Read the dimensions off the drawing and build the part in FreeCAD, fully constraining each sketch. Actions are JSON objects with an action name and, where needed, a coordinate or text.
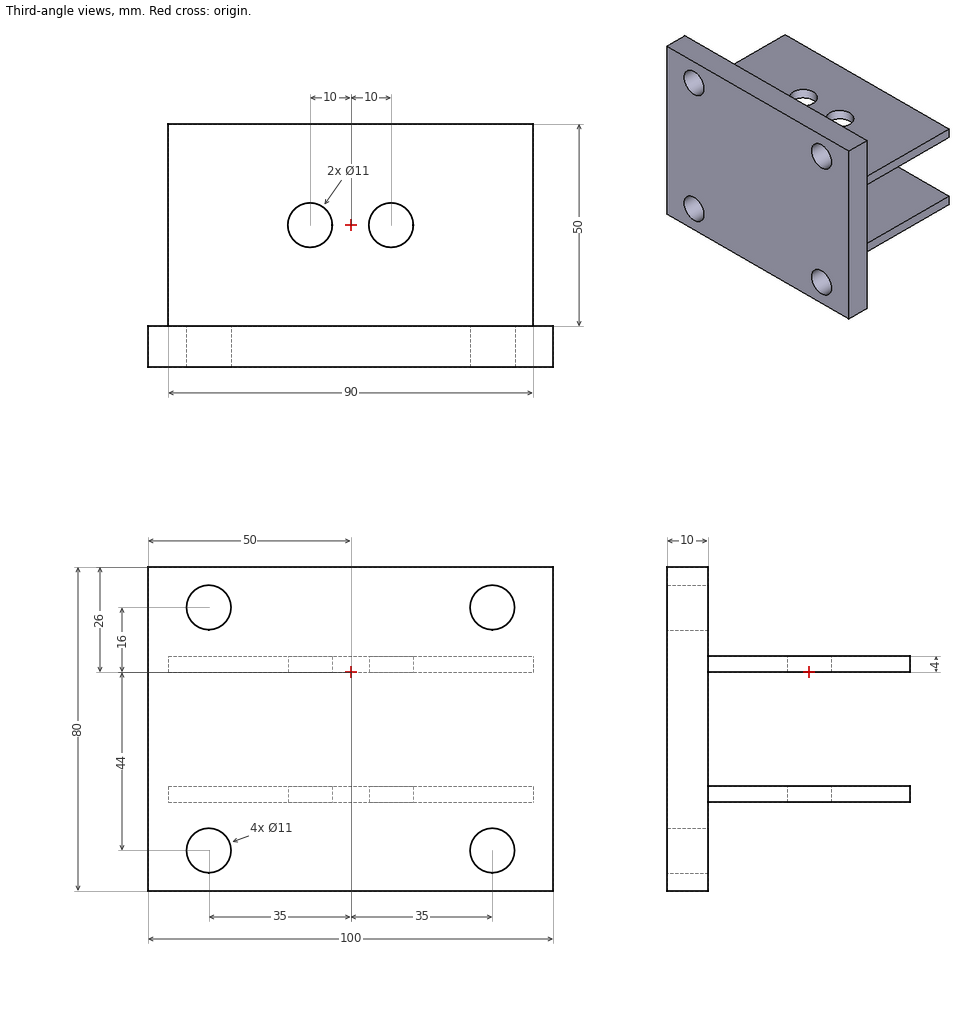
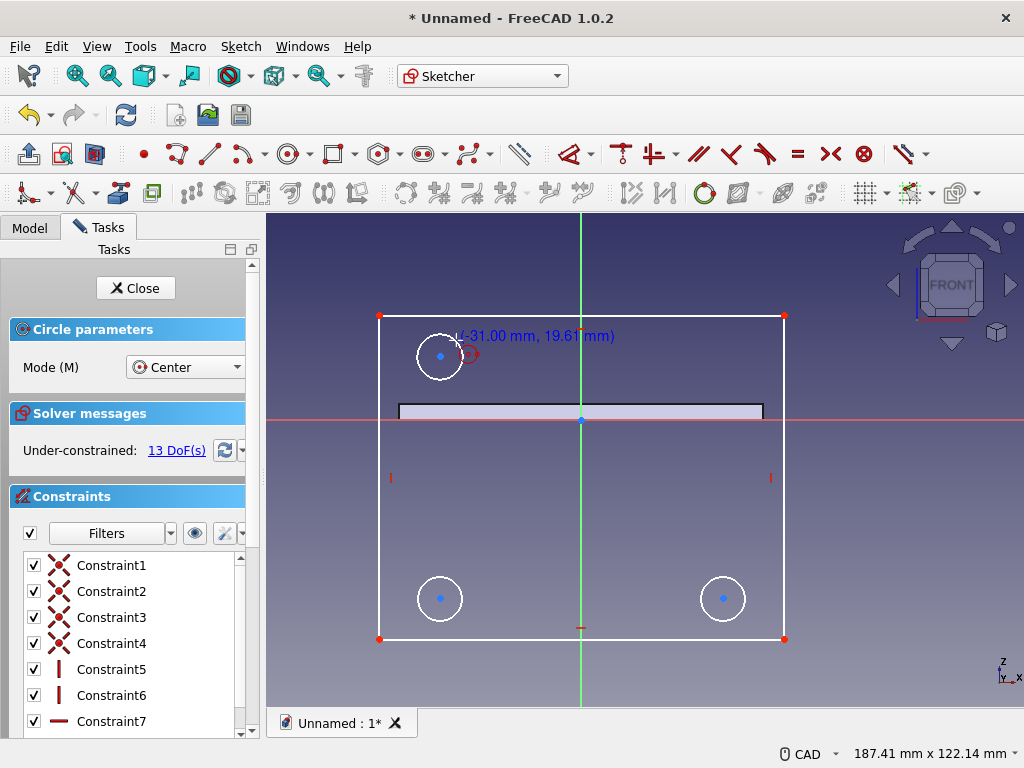
{"action": "left_click", "coordinate": [723, 356]}
{"action": "left_click", "coordinate": [739, 340]}
{"action": "key", "text": "Escape"}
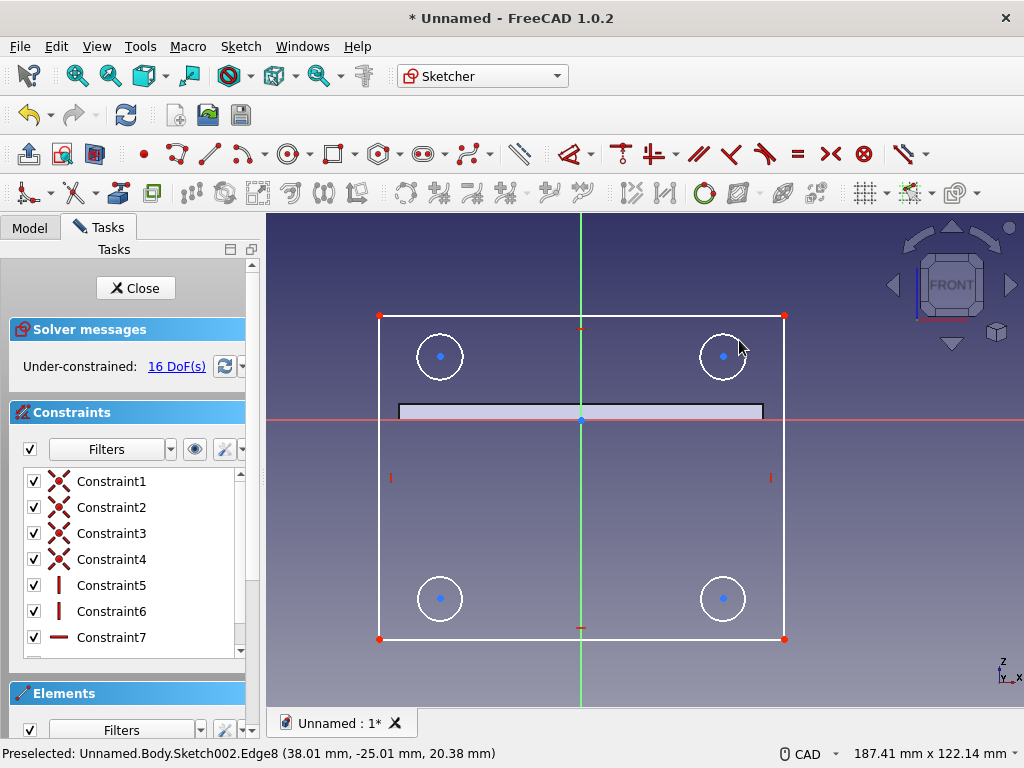
{"action": "left_click", "coordinate": [455, 583]}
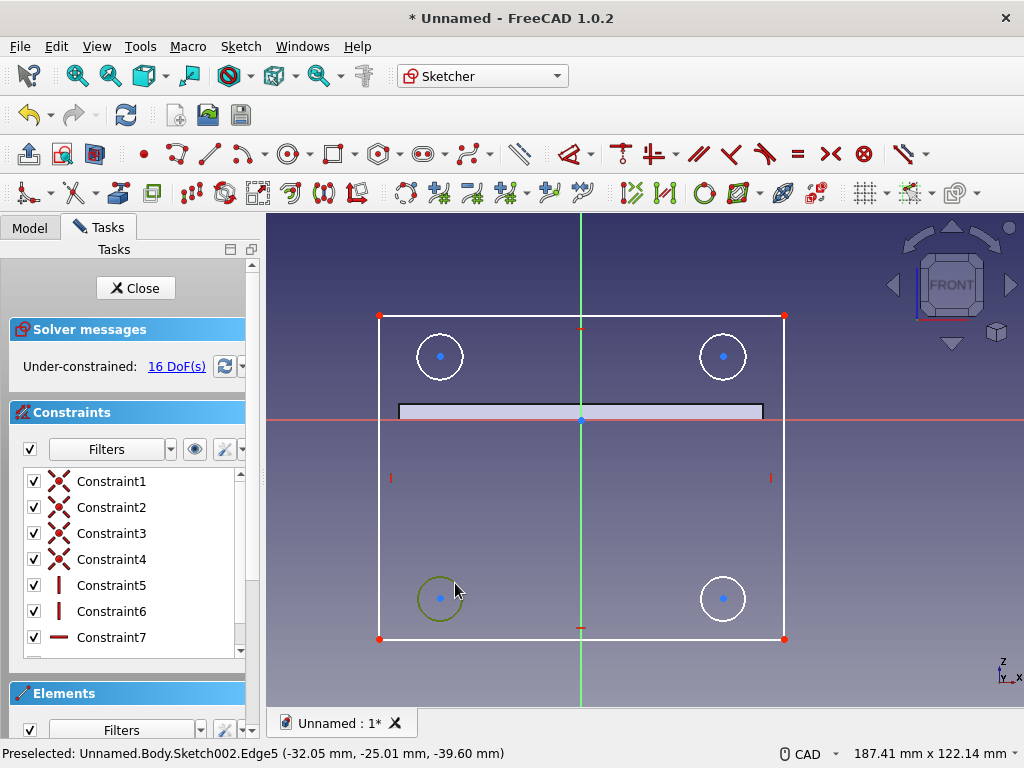
{"action": "left_click", "coordinate": [738, 583]}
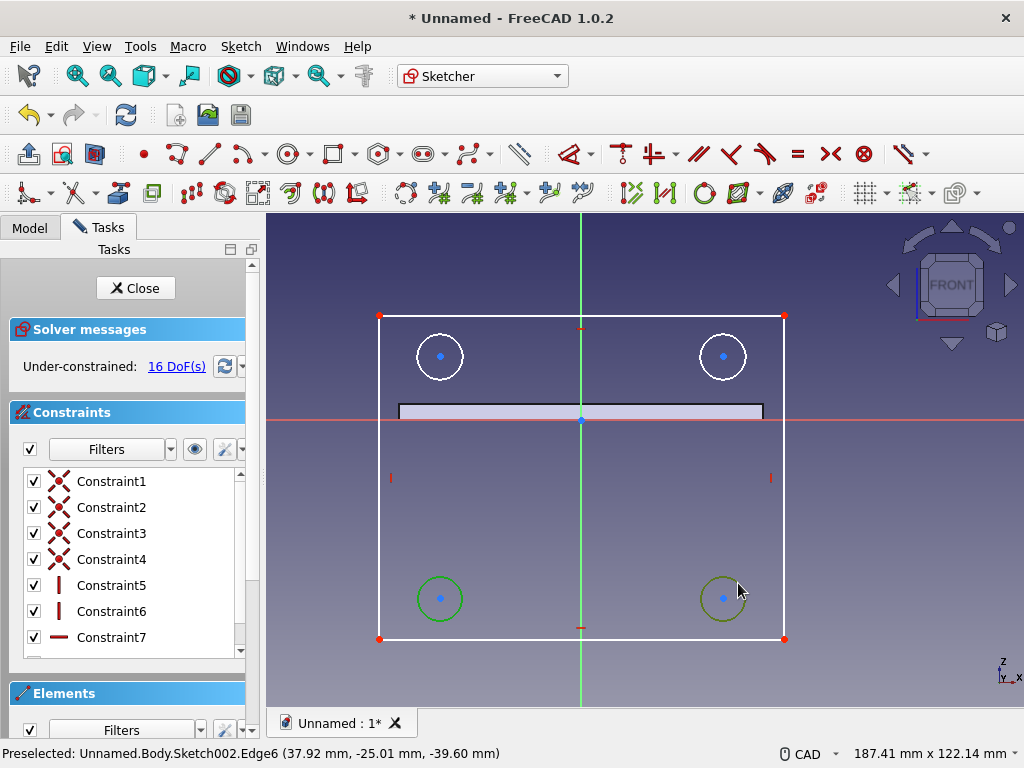
{"action": "left_click", "coordinate": [456, 341]}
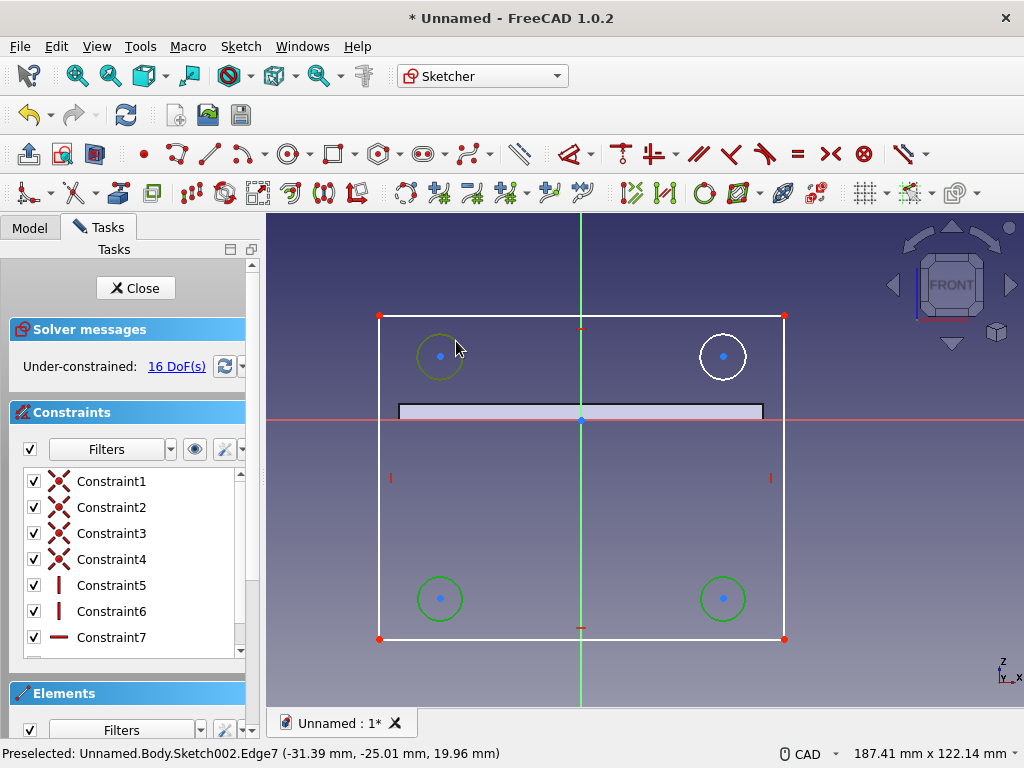
{"action": "left_click", "coordinate": [739, 341]}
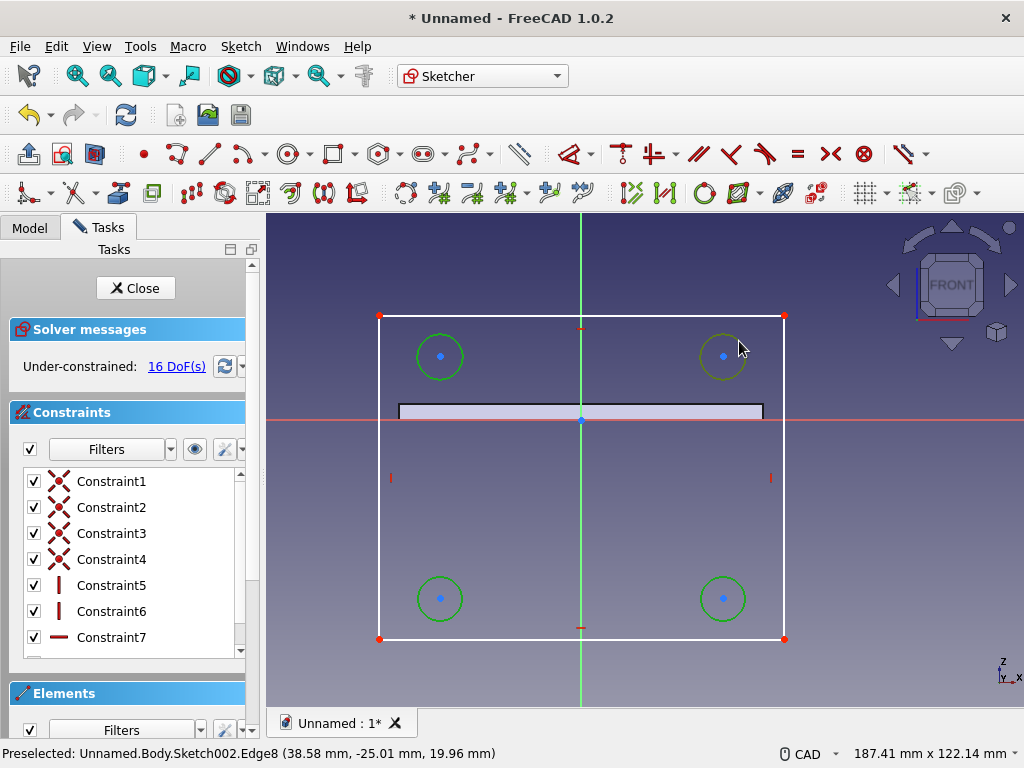
{"action": "key", "text": "e"}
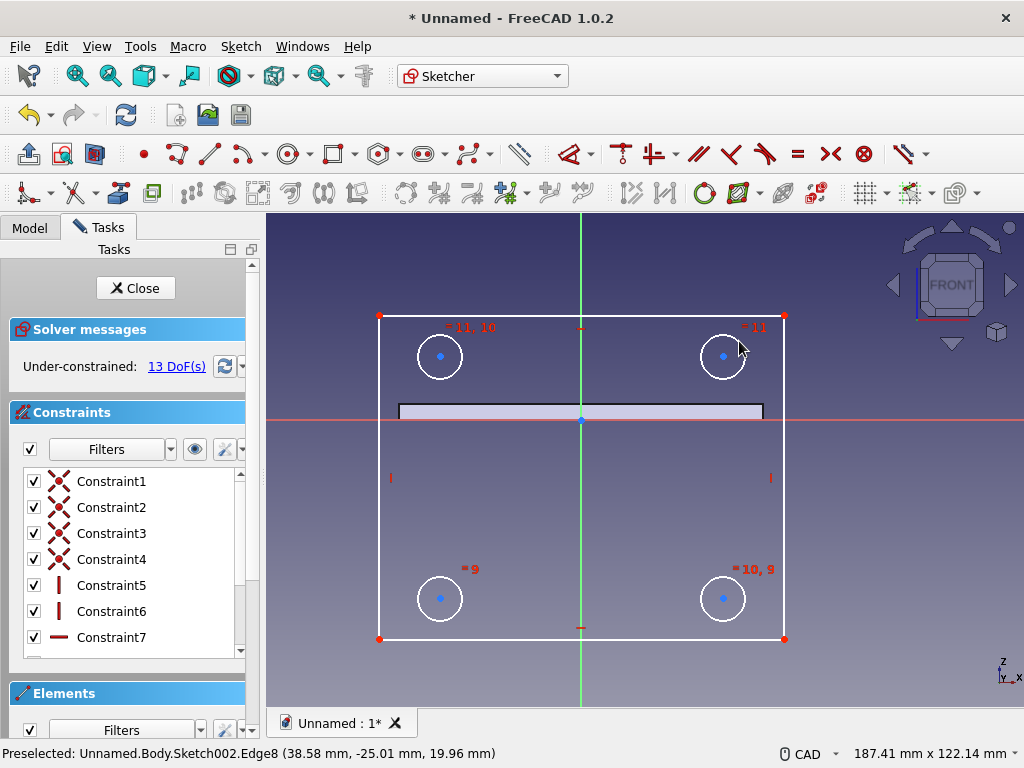
{"action": "left_click", "coordinate": [440, 599]}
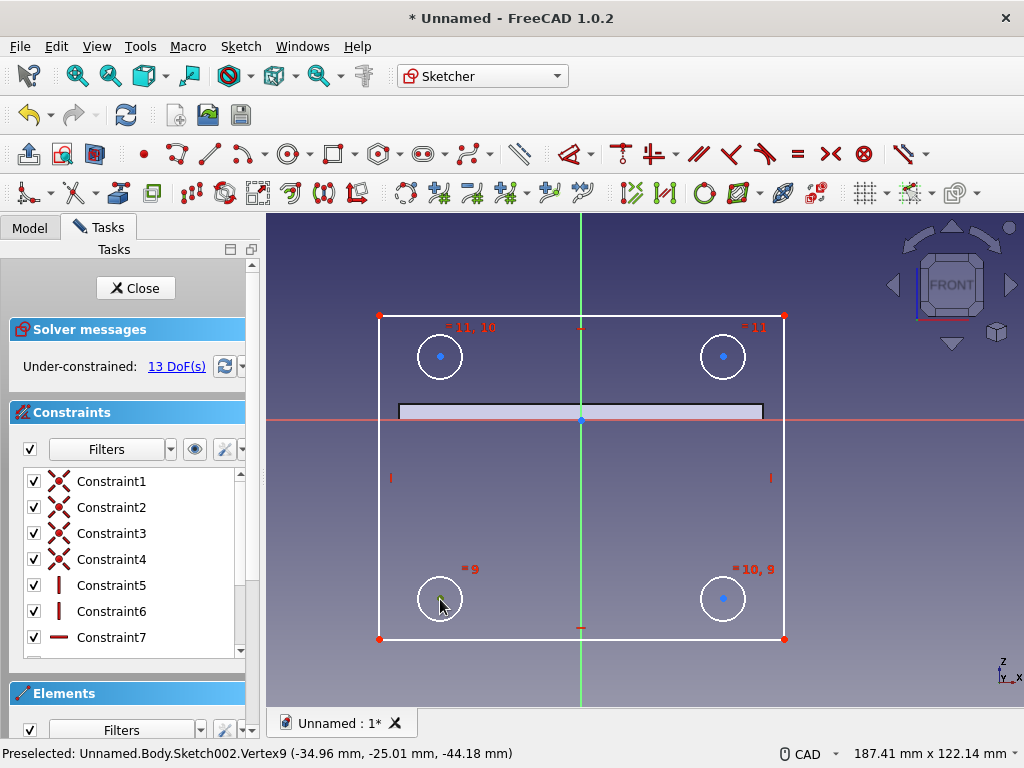
{"action": "left_click", "coordinate": [723, 599]}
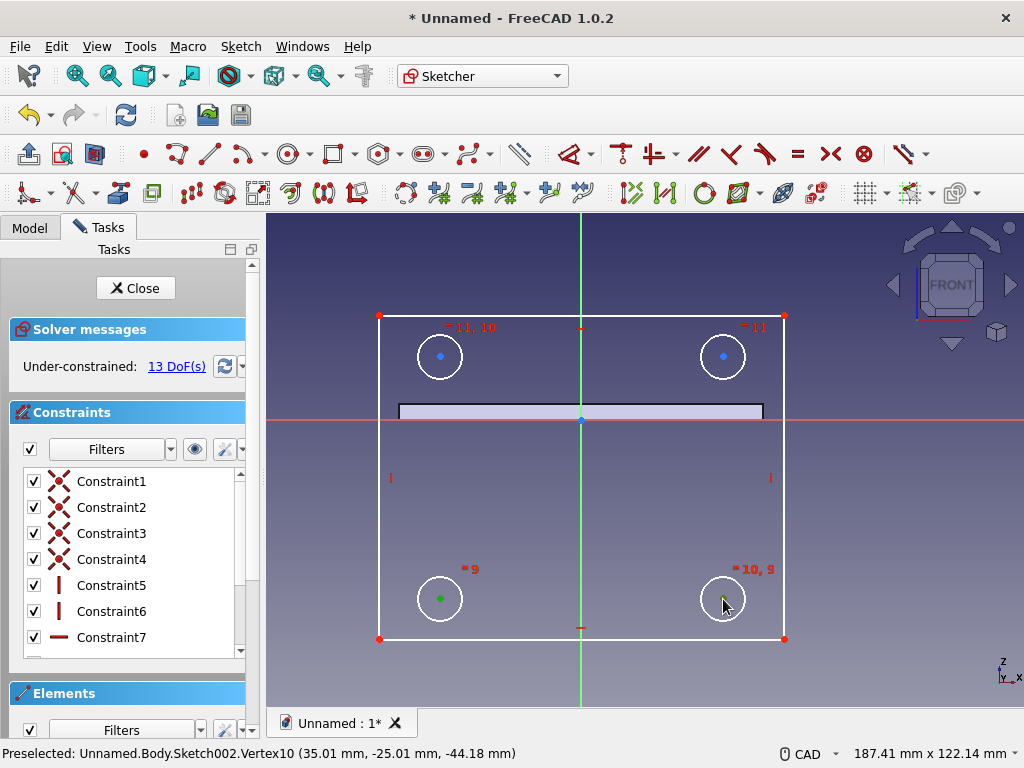
{"action": "key", "text": "h"}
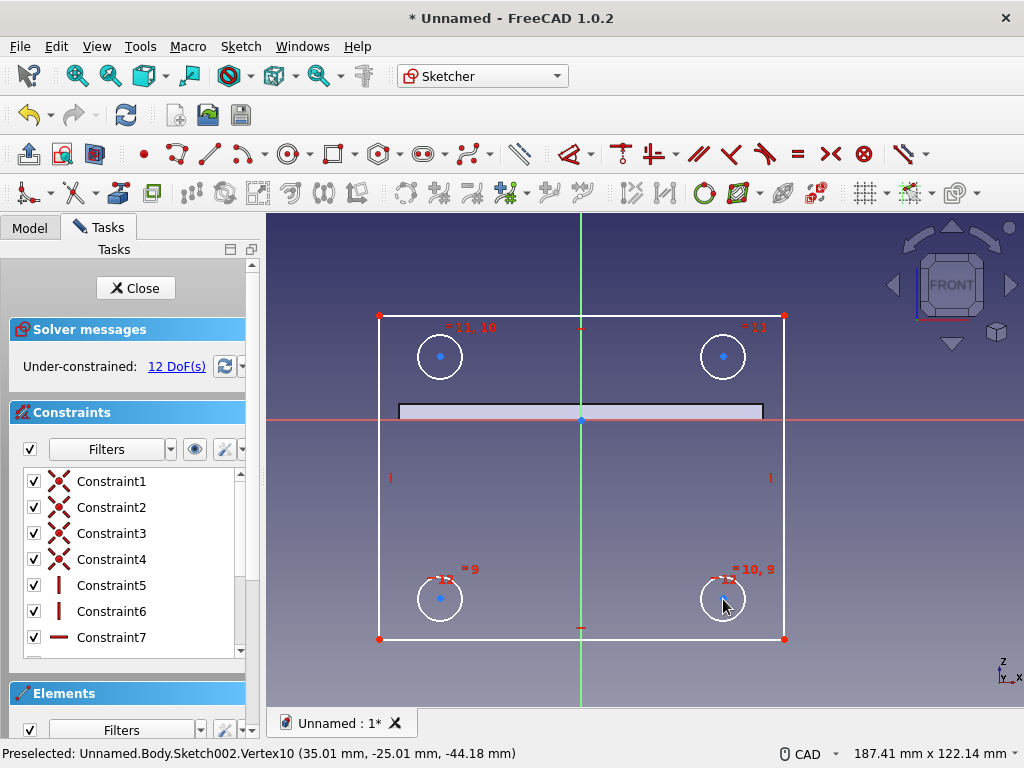
{"action": "left_click", "coordinate": [440, 599]}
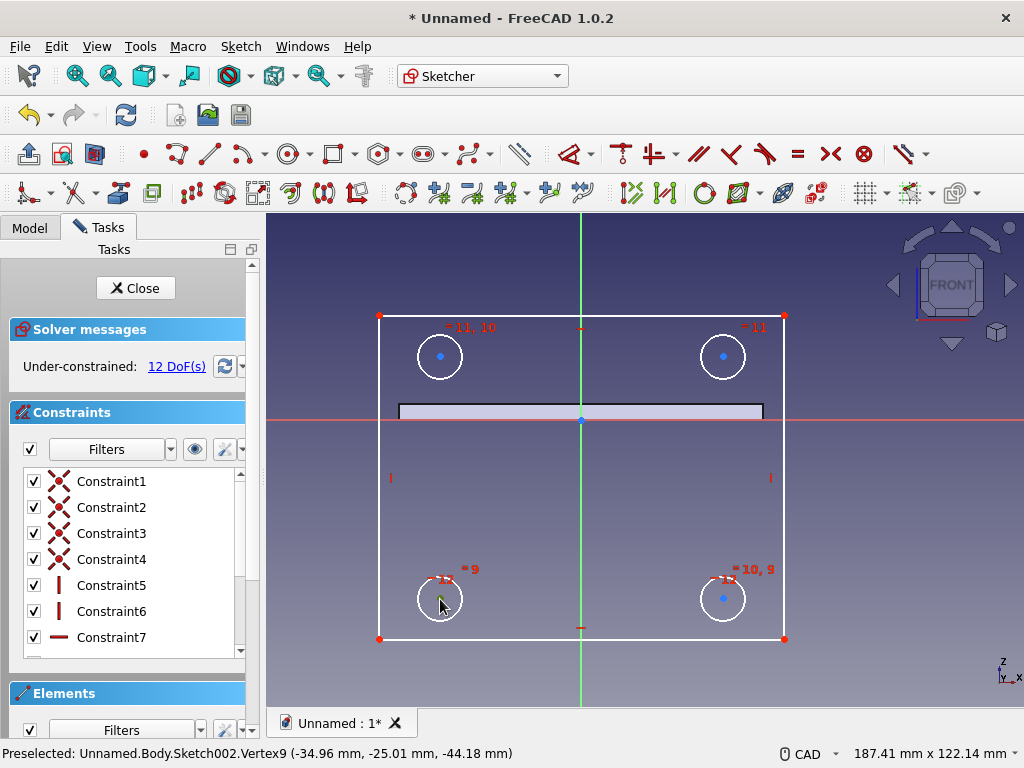
{"action": "left_click", "coordinate": [440, 357]}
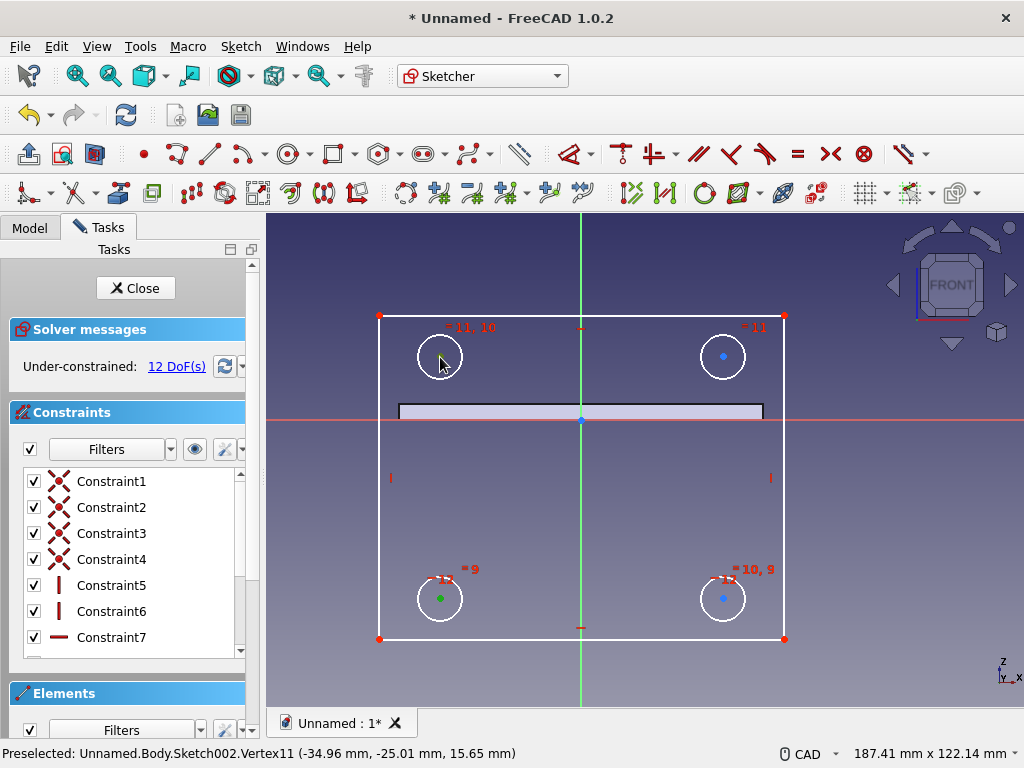
{"action": "left_click", "coordinate": [676, 154]}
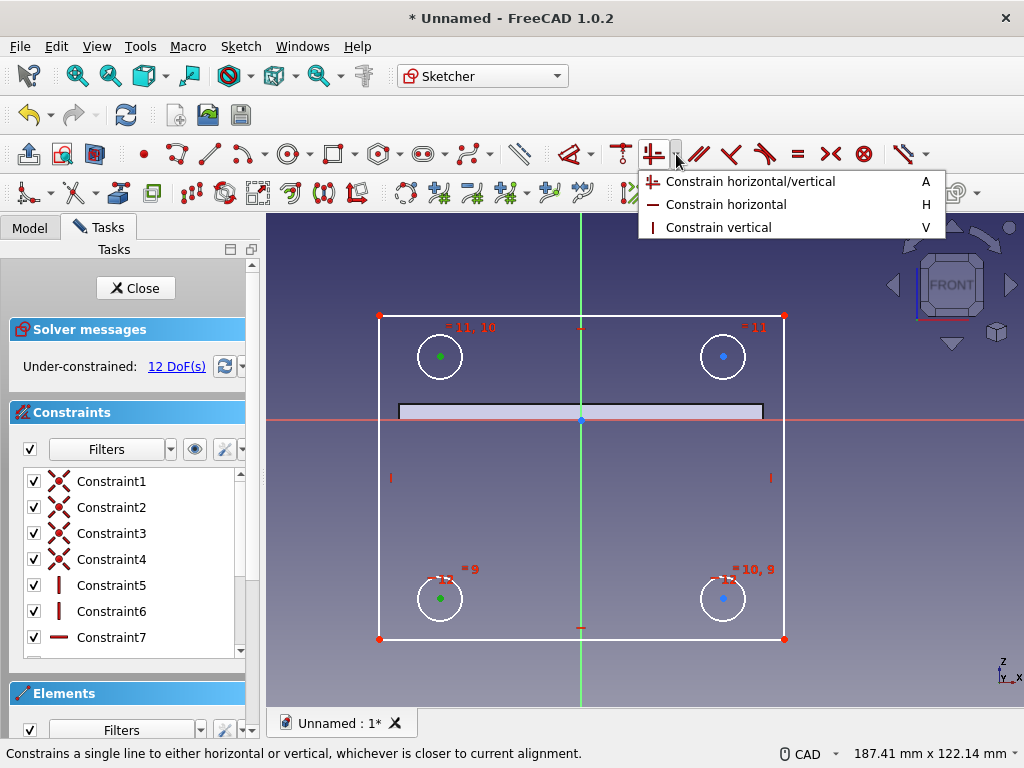
{"action": "left_click", "coordinate": [792, 228]}